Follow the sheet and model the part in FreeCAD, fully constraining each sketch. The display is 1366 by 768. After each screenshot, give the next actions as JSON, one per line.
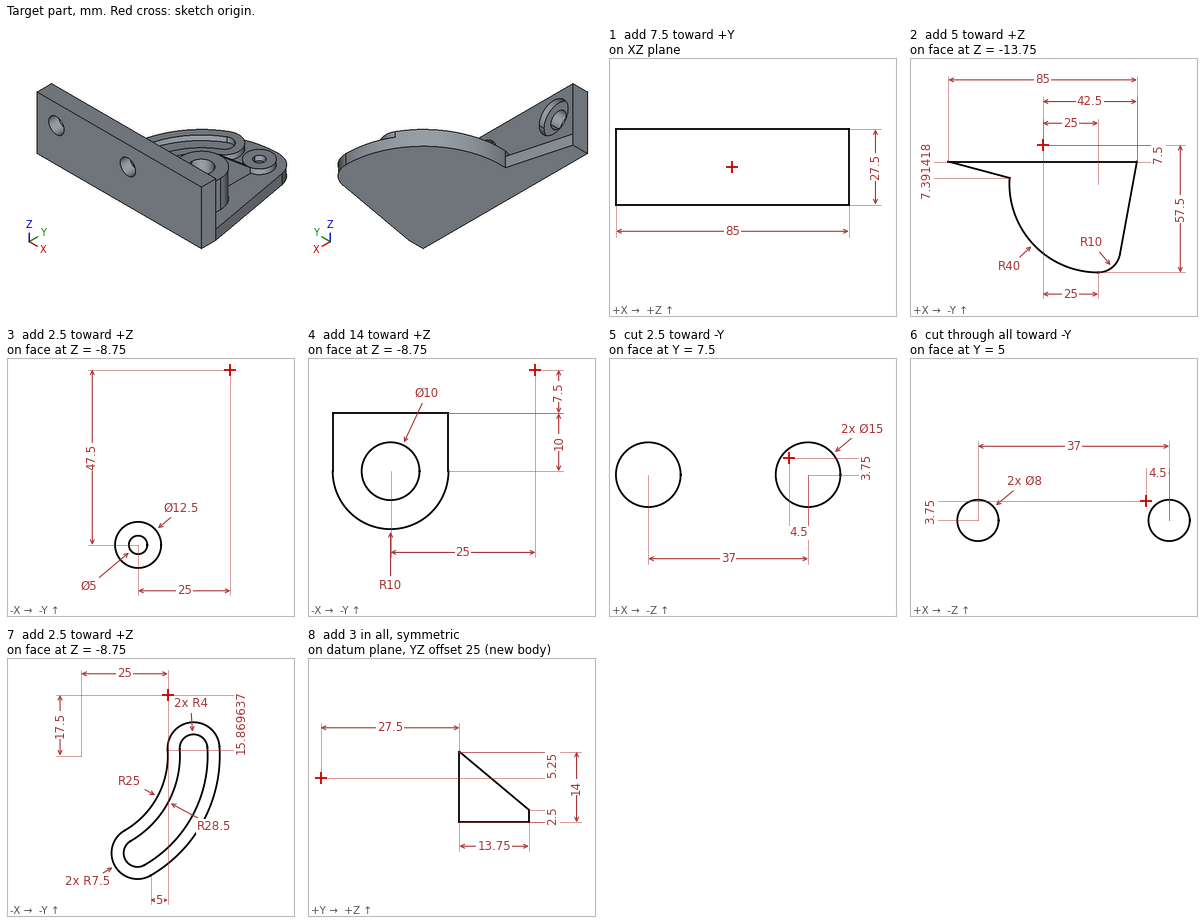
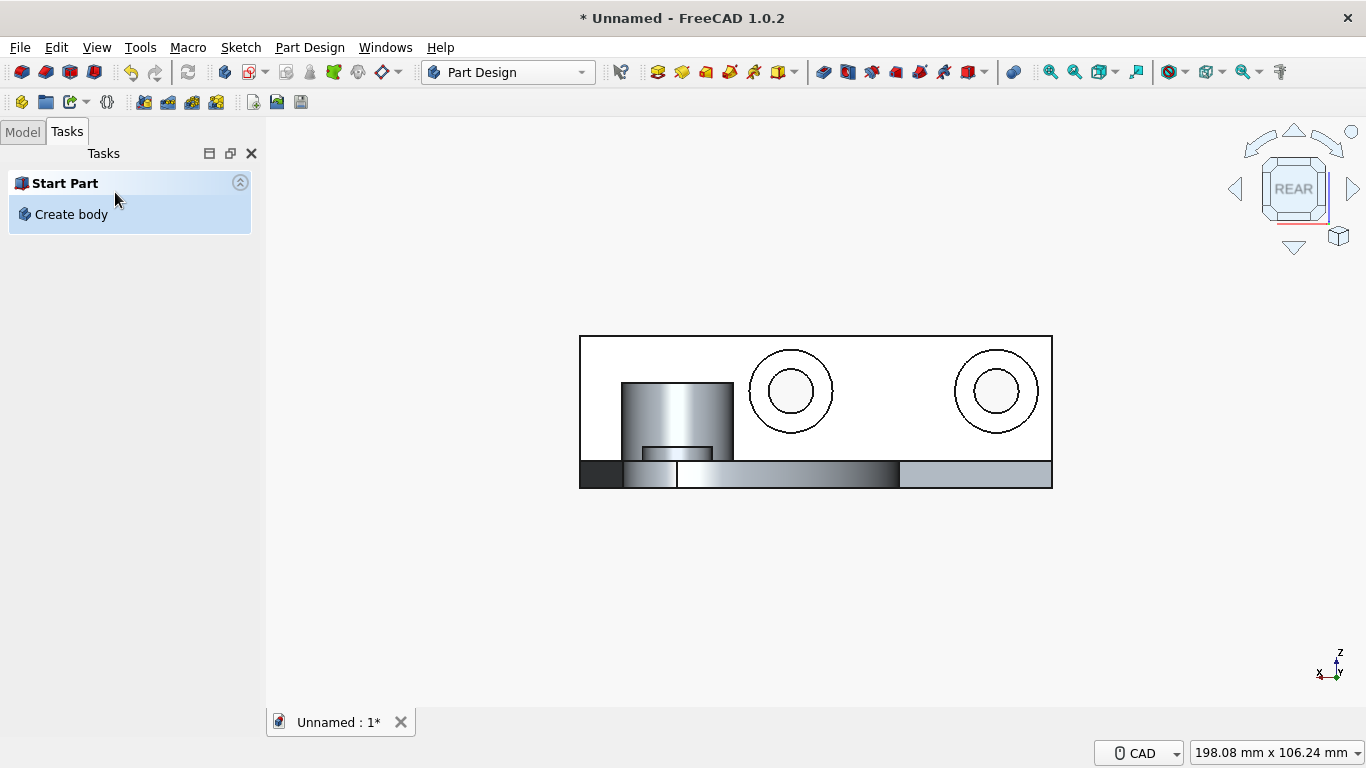
{"action": "left_click", "coordinate": [1052, 72]}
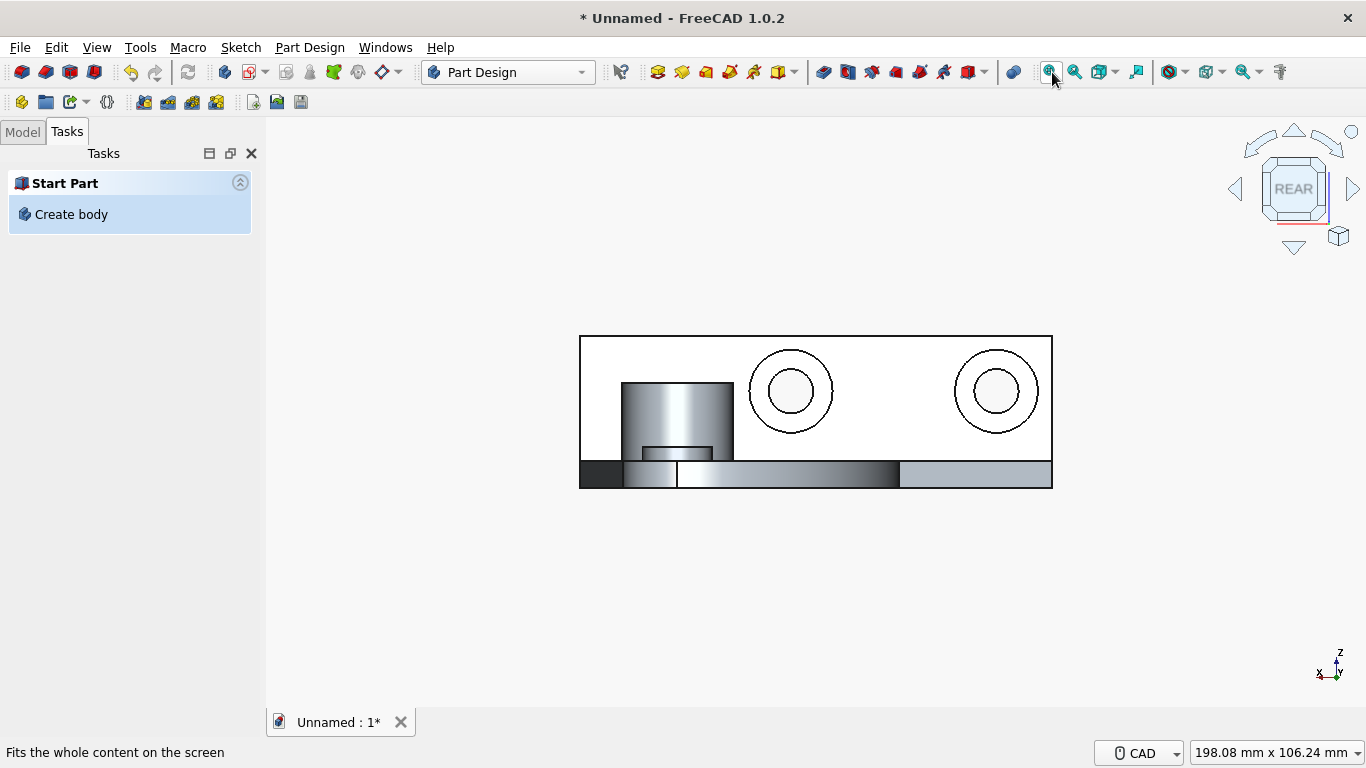
{"action": "key", "text": "0"}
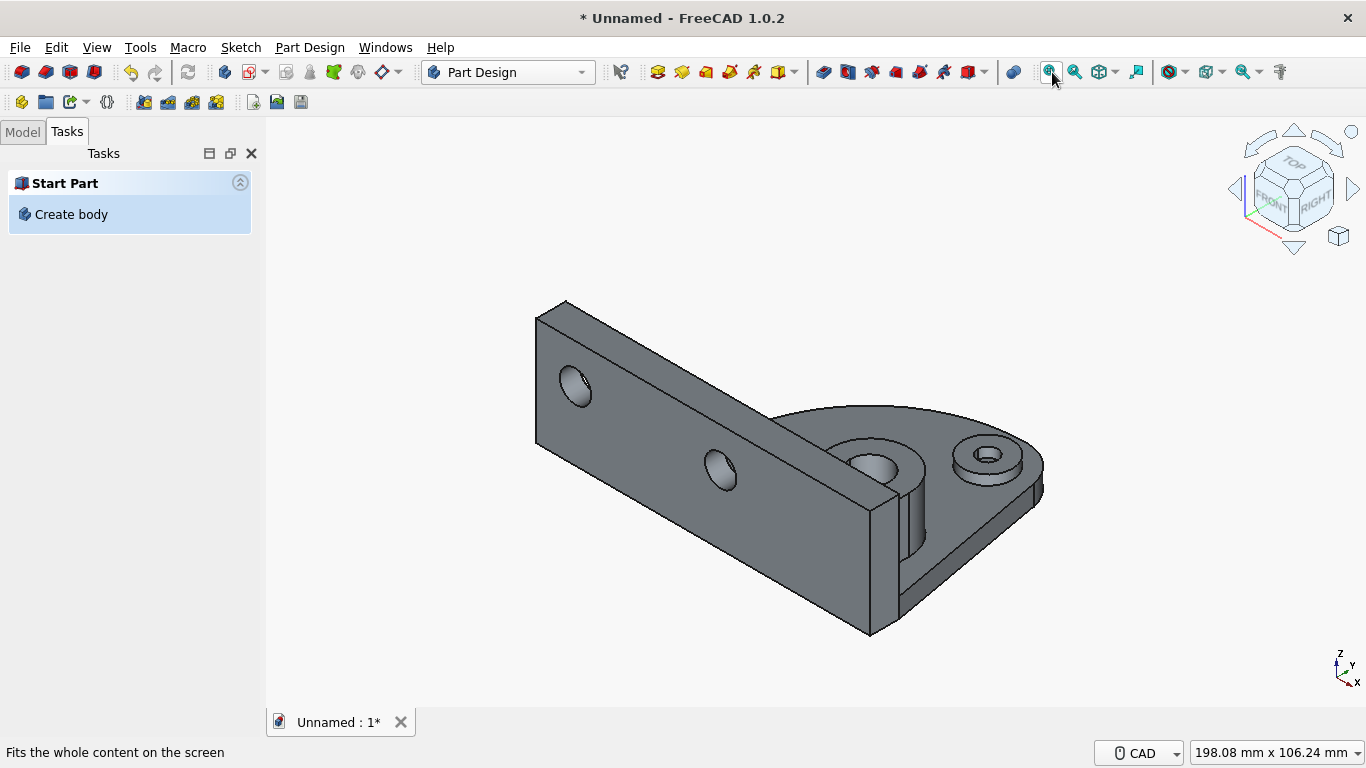
{"action": "left_click", "coordinate": [935, 437]}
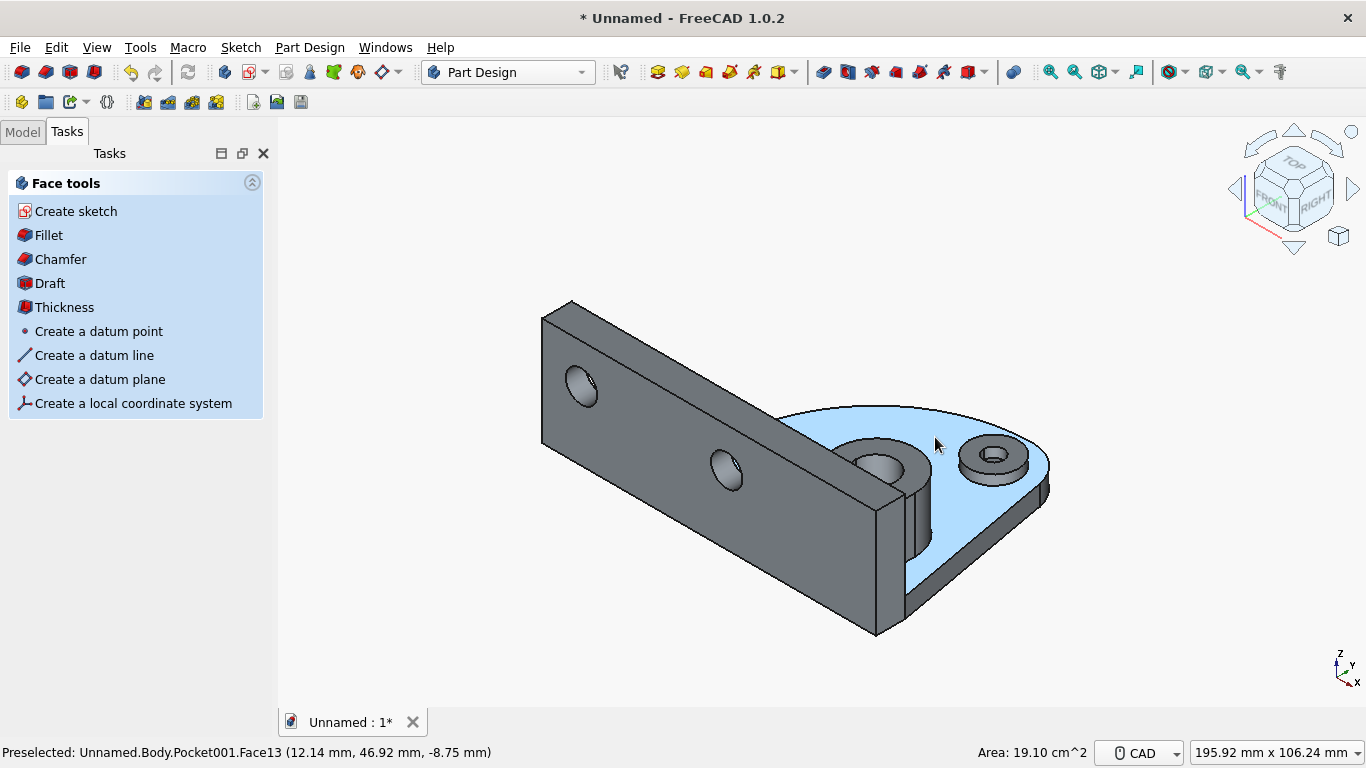
{"action": "left_click", "coordinate": [250, 72]}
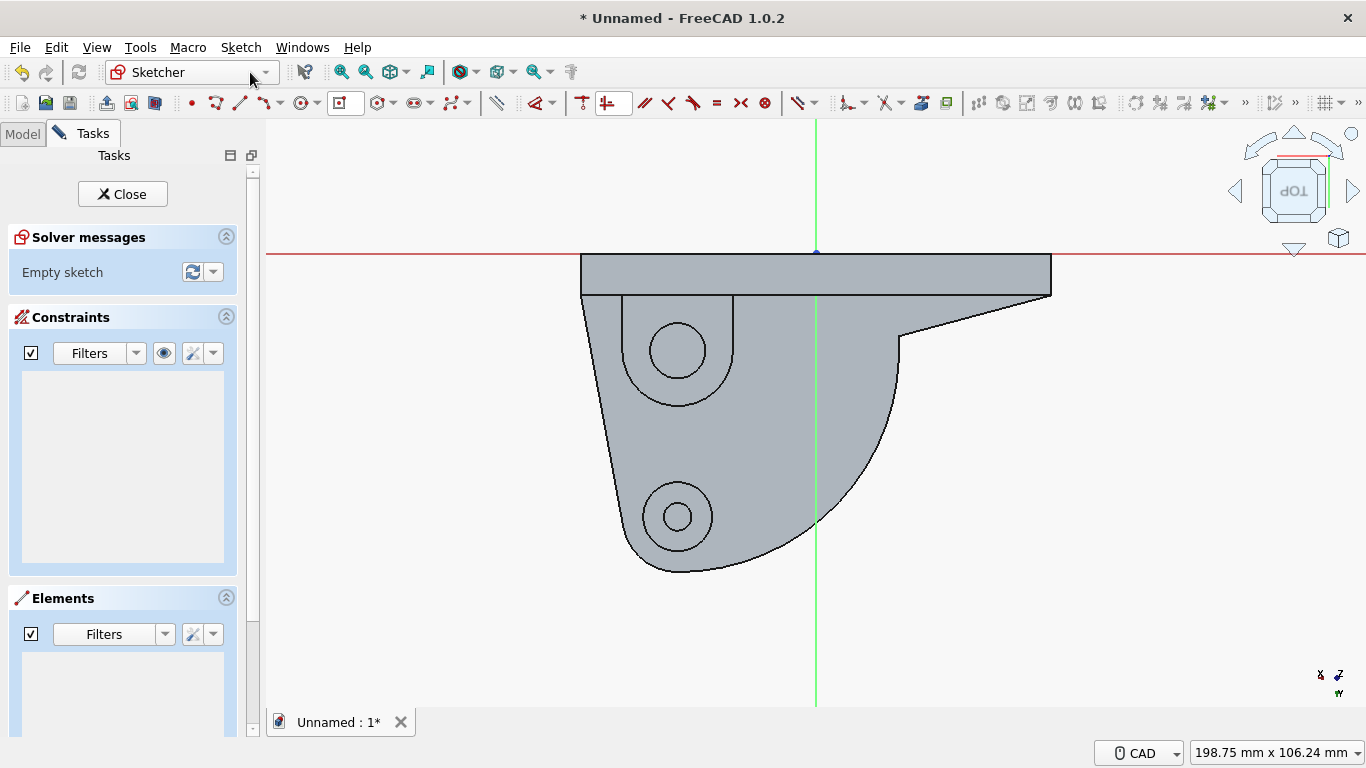
{"action": "left_click", "coordinate": [264, 104]}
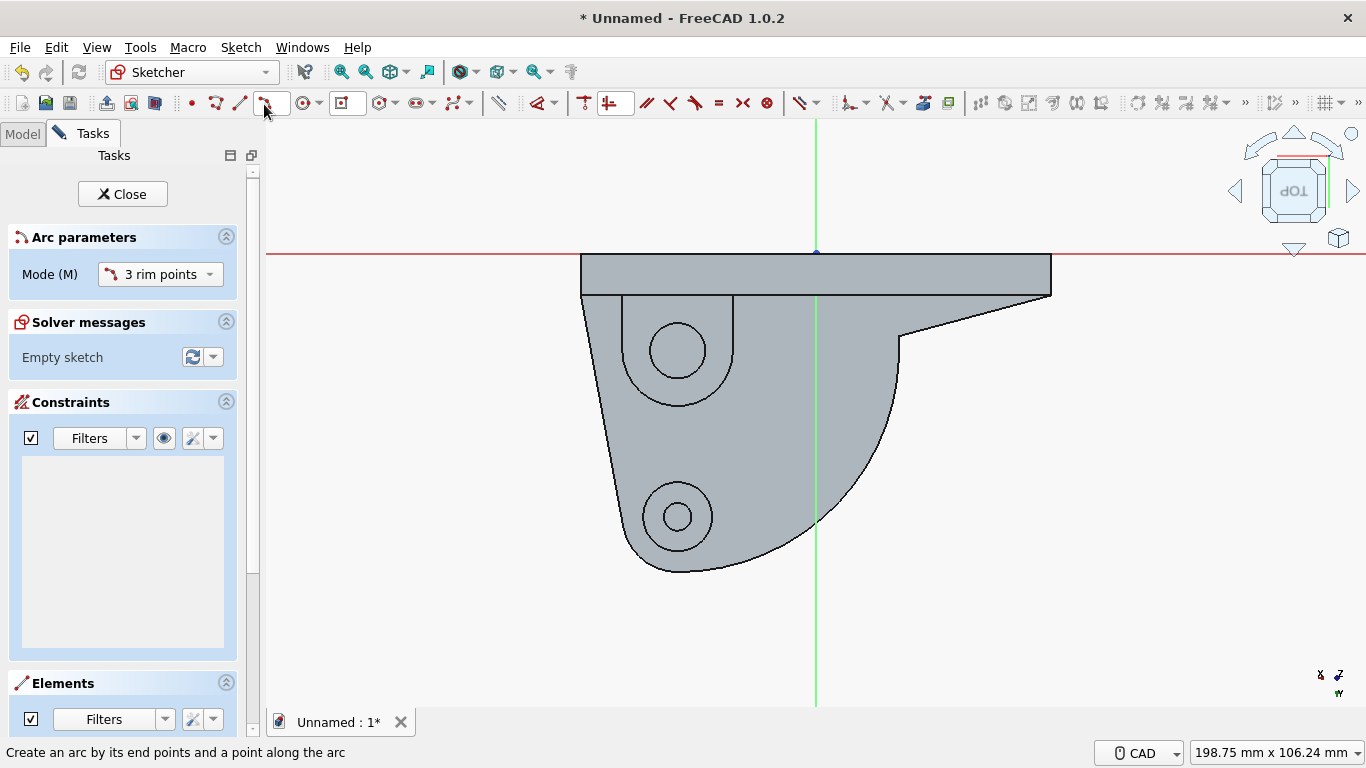
{"action": "scroll", "coordinate": [816, 342], "scroll_direction": "up", "scroll_amount": 20}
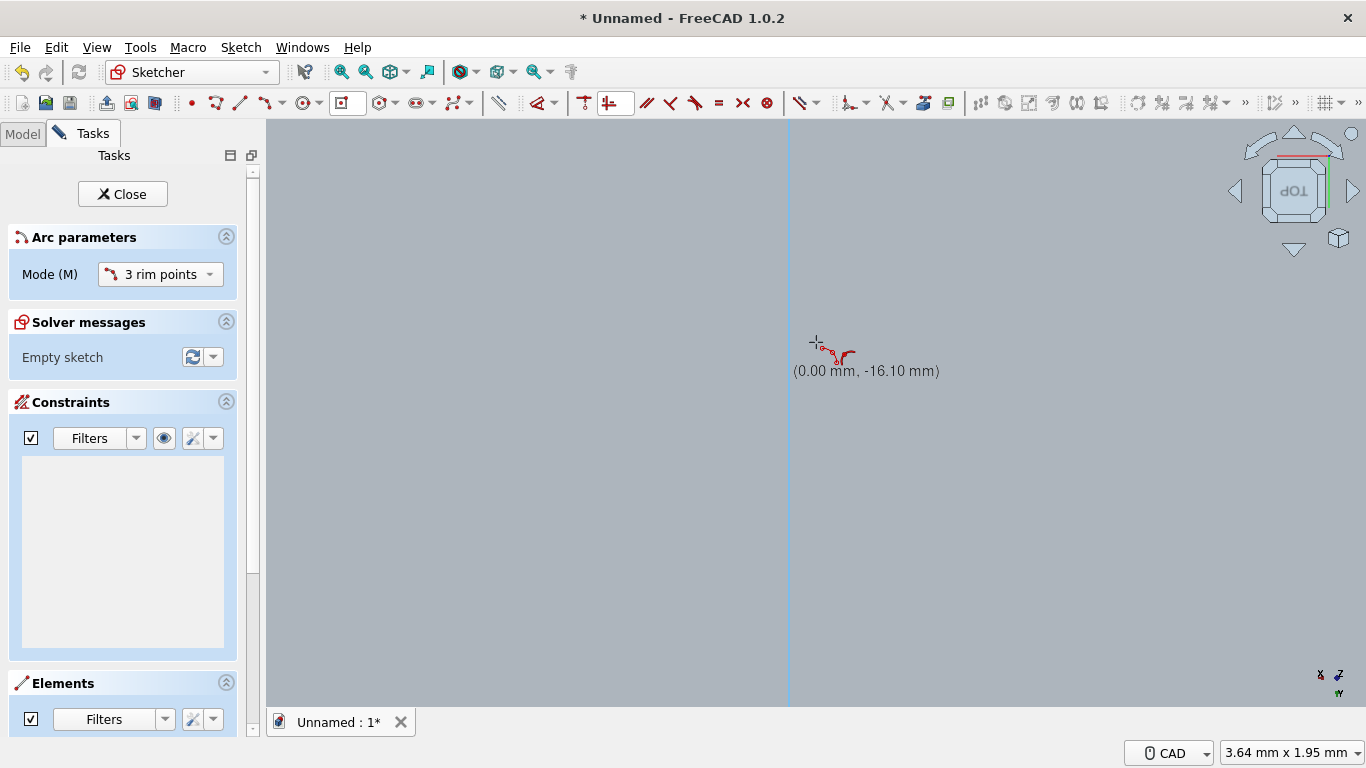
{"action": "left_click", "coordinate": [773, 306]}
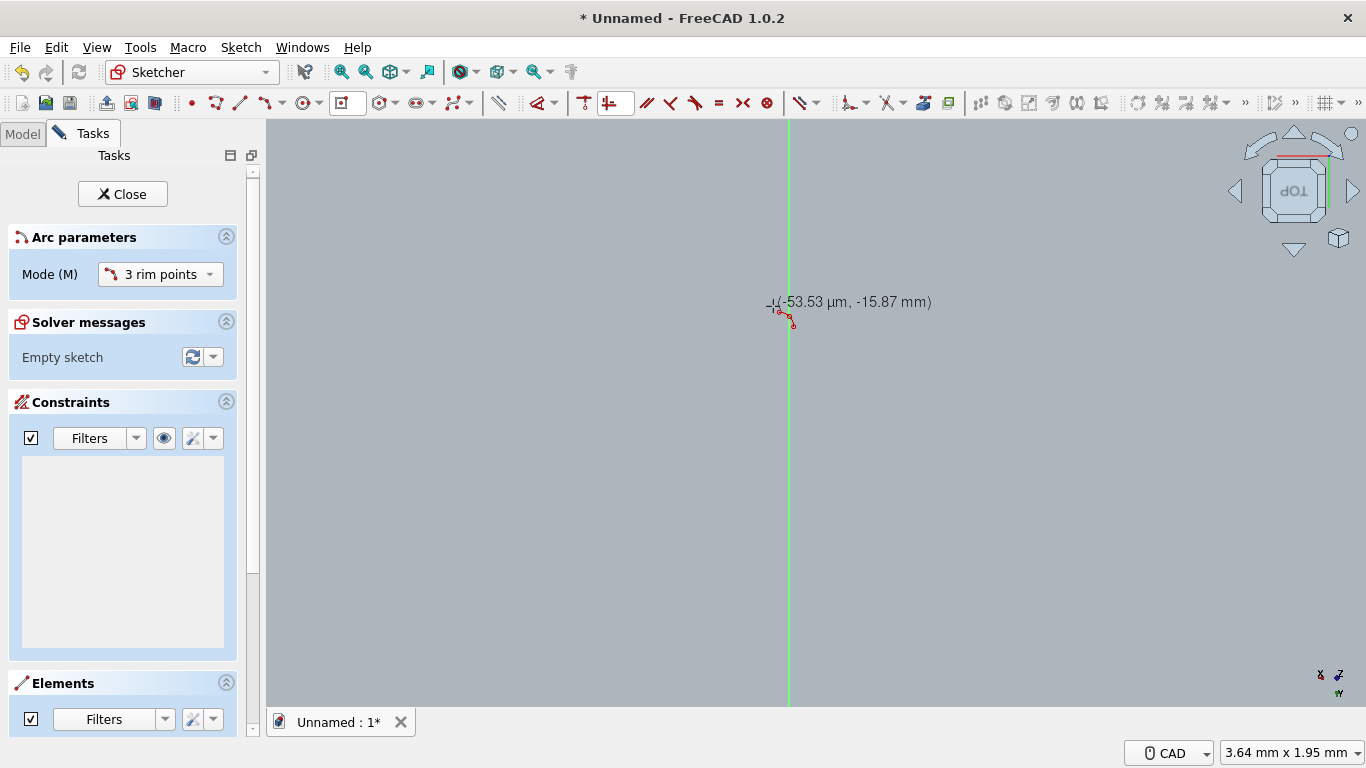
{"action": "scroll", "coordinate": [748, 329], "scroll_direction": "down", "scroll_amount": 18}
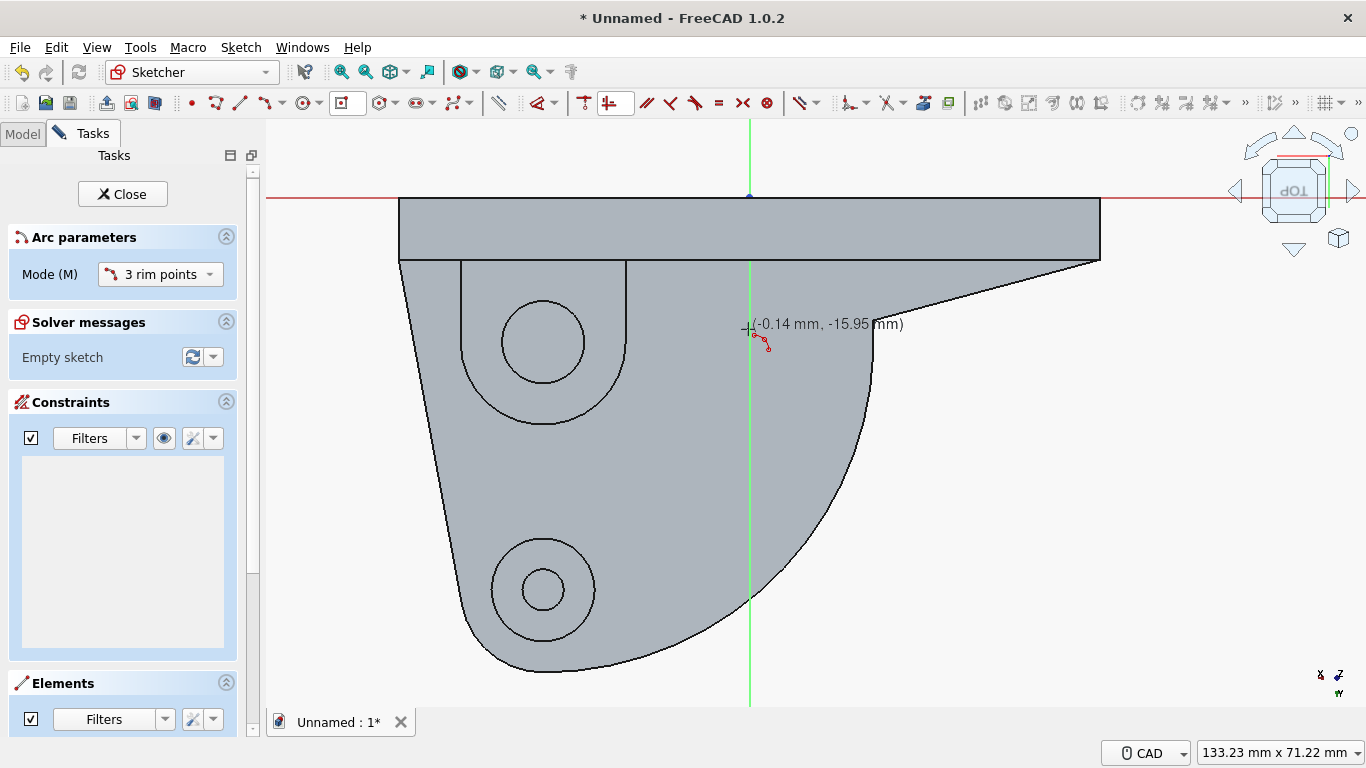
{"action": "left_click", "coordinate": [646, 521]}
{"action": "left_click", "coordinate": [725, 440]}